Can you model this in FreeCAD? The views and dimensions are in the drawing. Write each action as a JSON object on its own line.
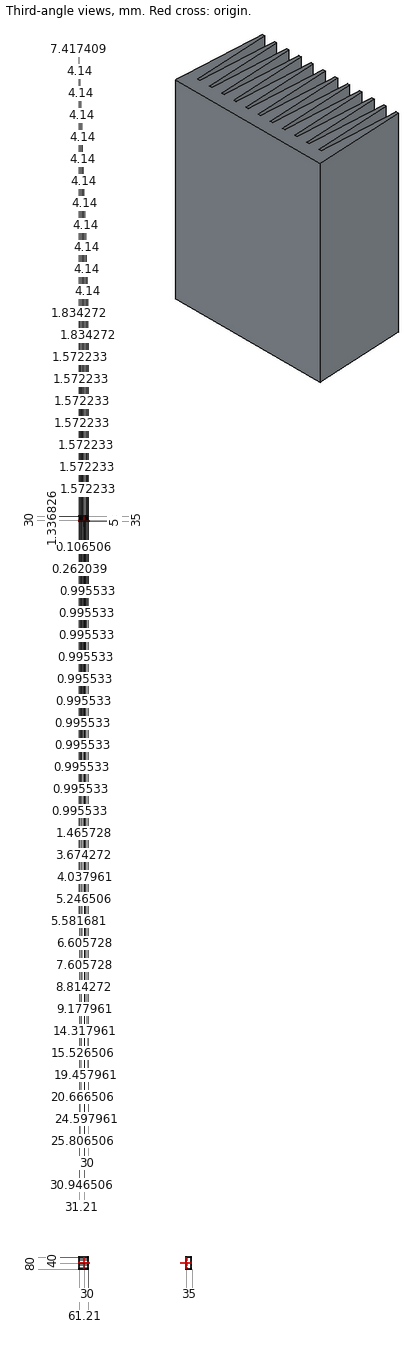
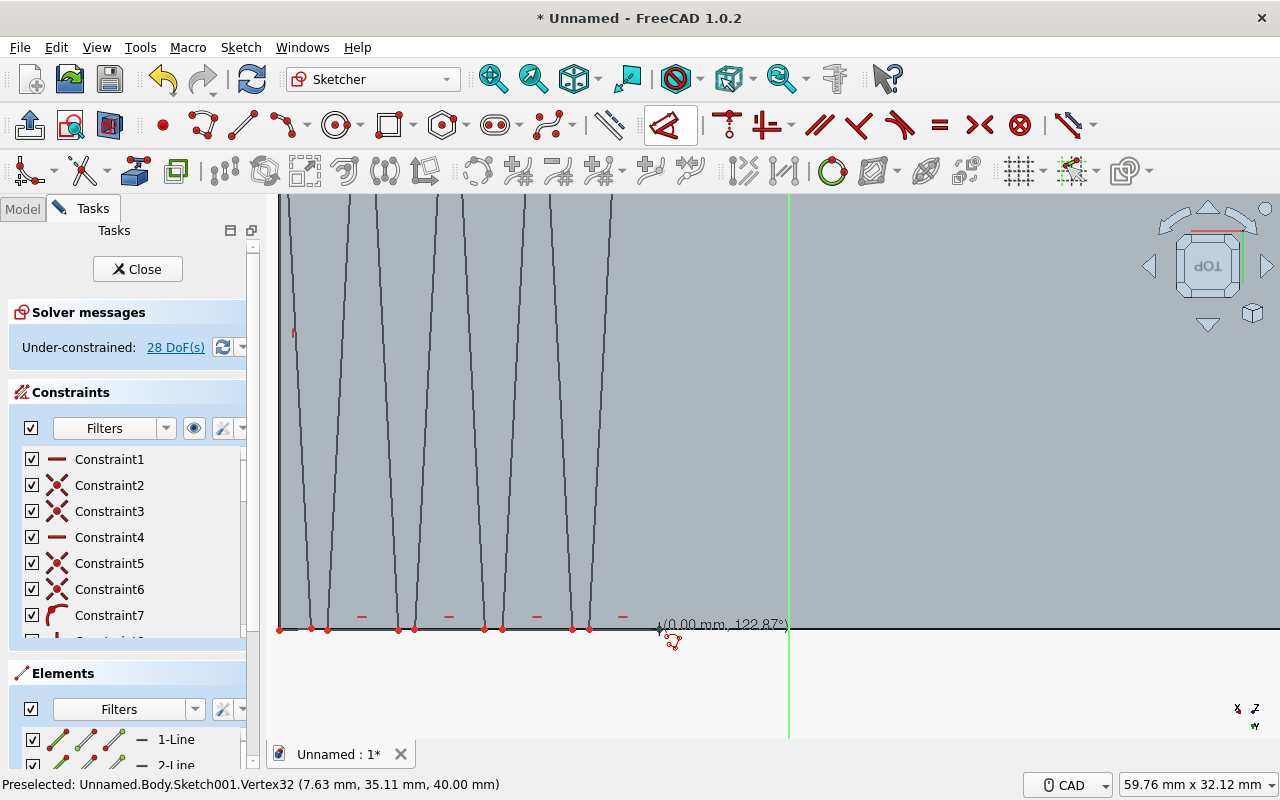
{"action": "scroll", "coordinate": [590, 630], "scroll_direction": "down", "scroll_amount": 3}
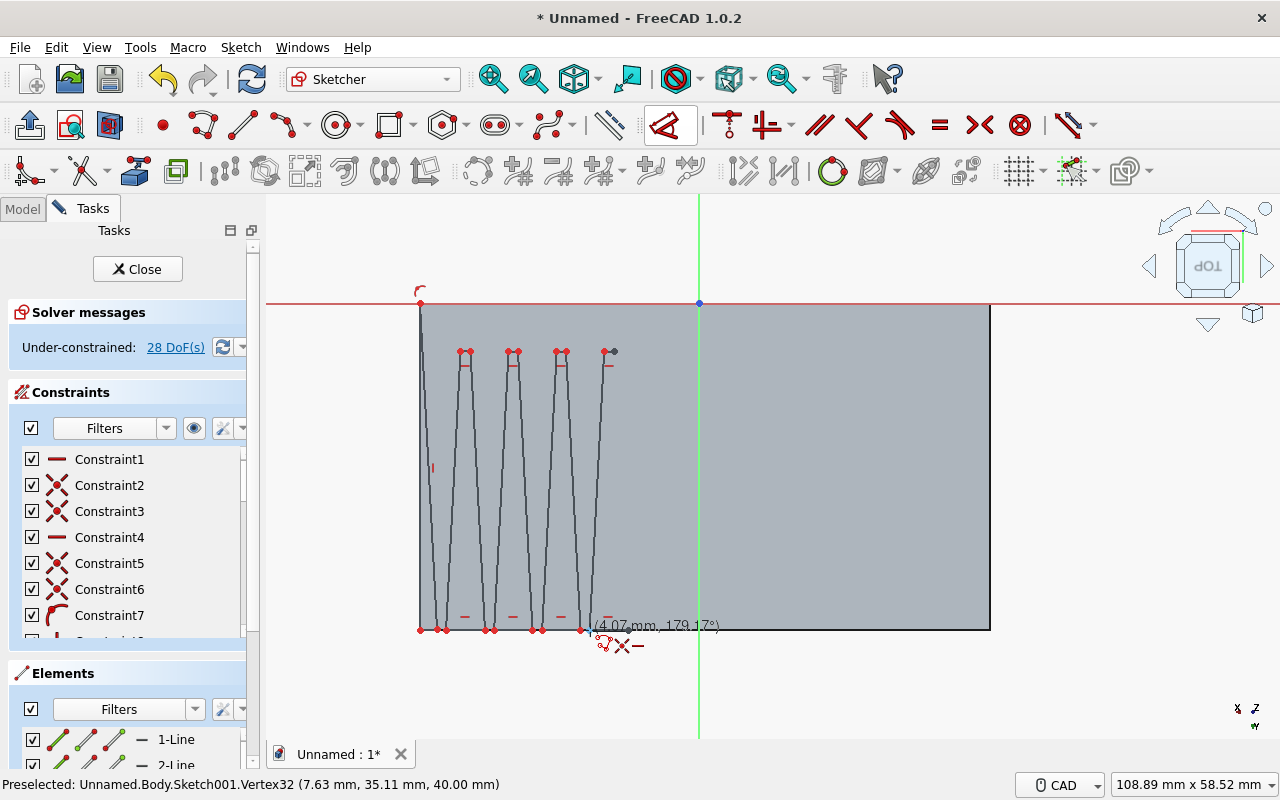
{"action": "scroll", "coordinate": [614, 351], "scroll_direction": "up", "scroll_amount": 7}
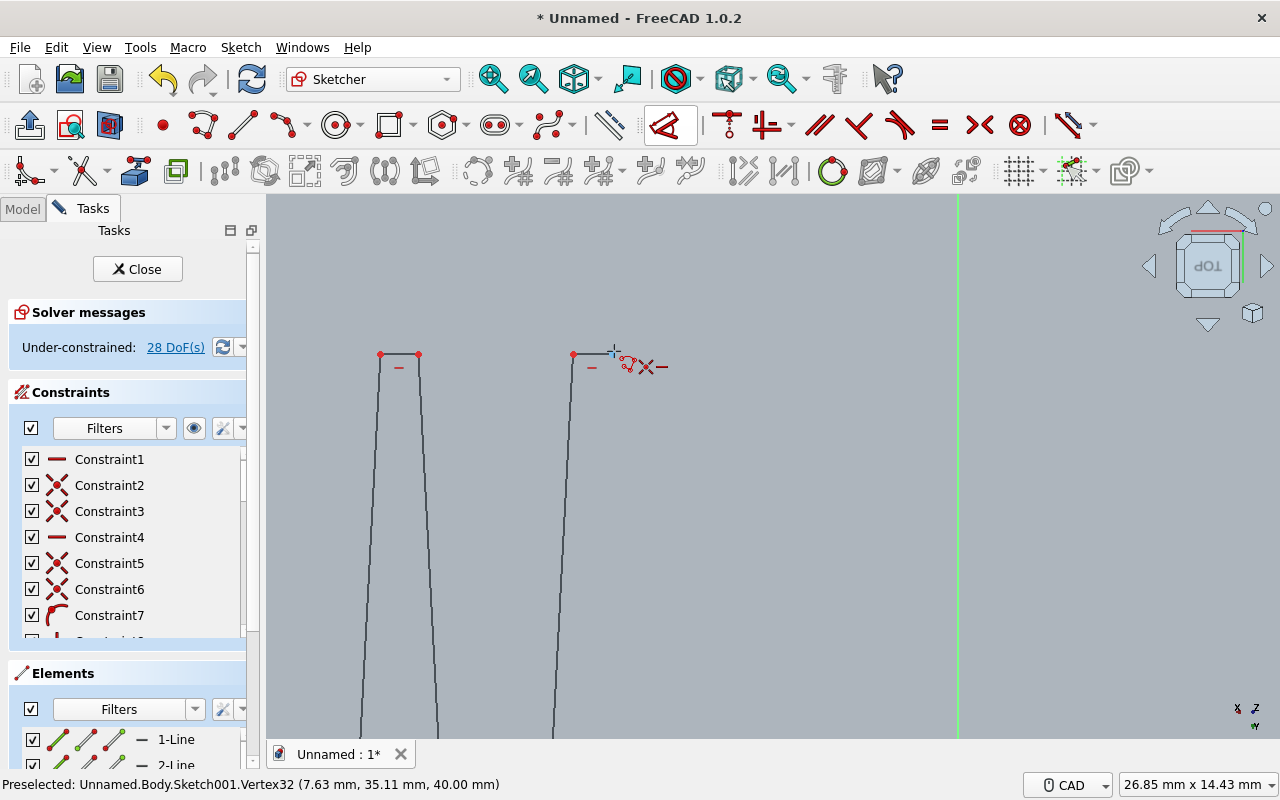
{"action": "left_click", "coordinate": [613, 354]}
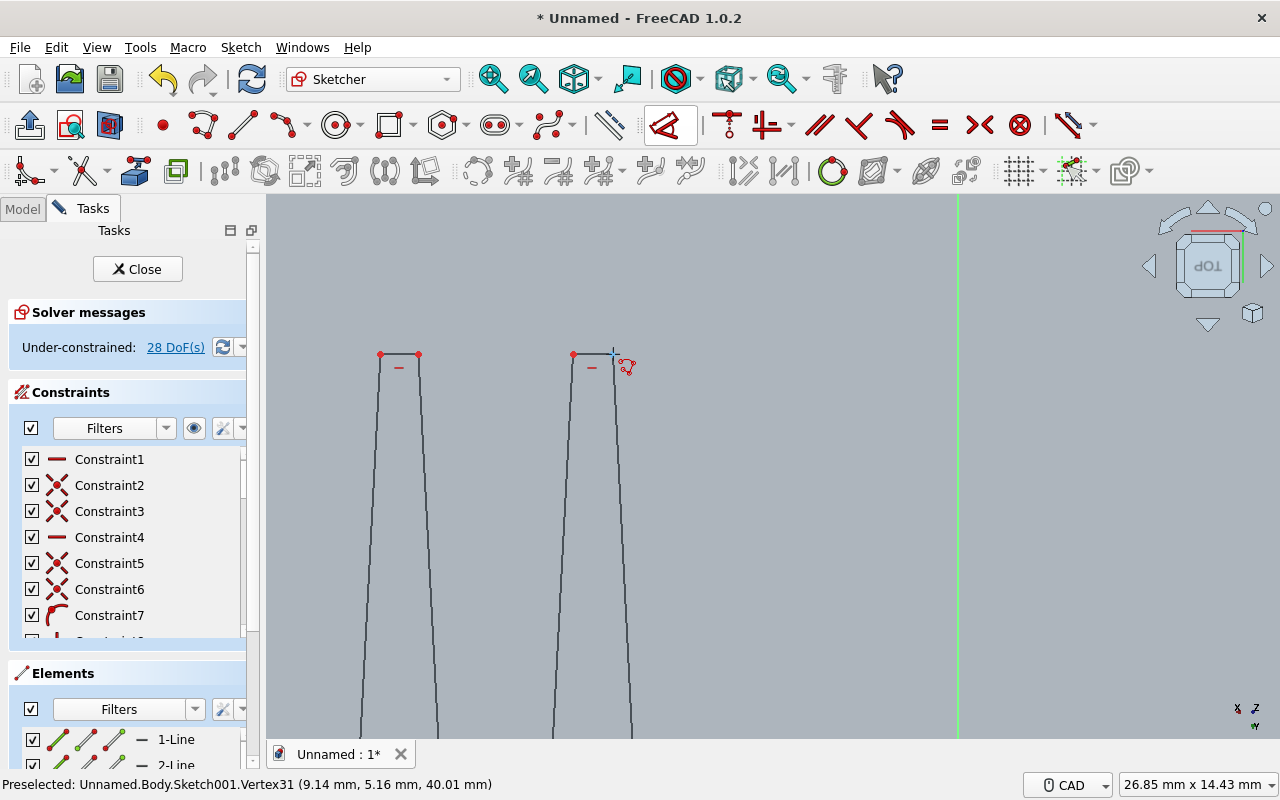
{"action": "scroll", "coordinate": [614, 351], "scroll_direction": "down", "scroll_amount": 7}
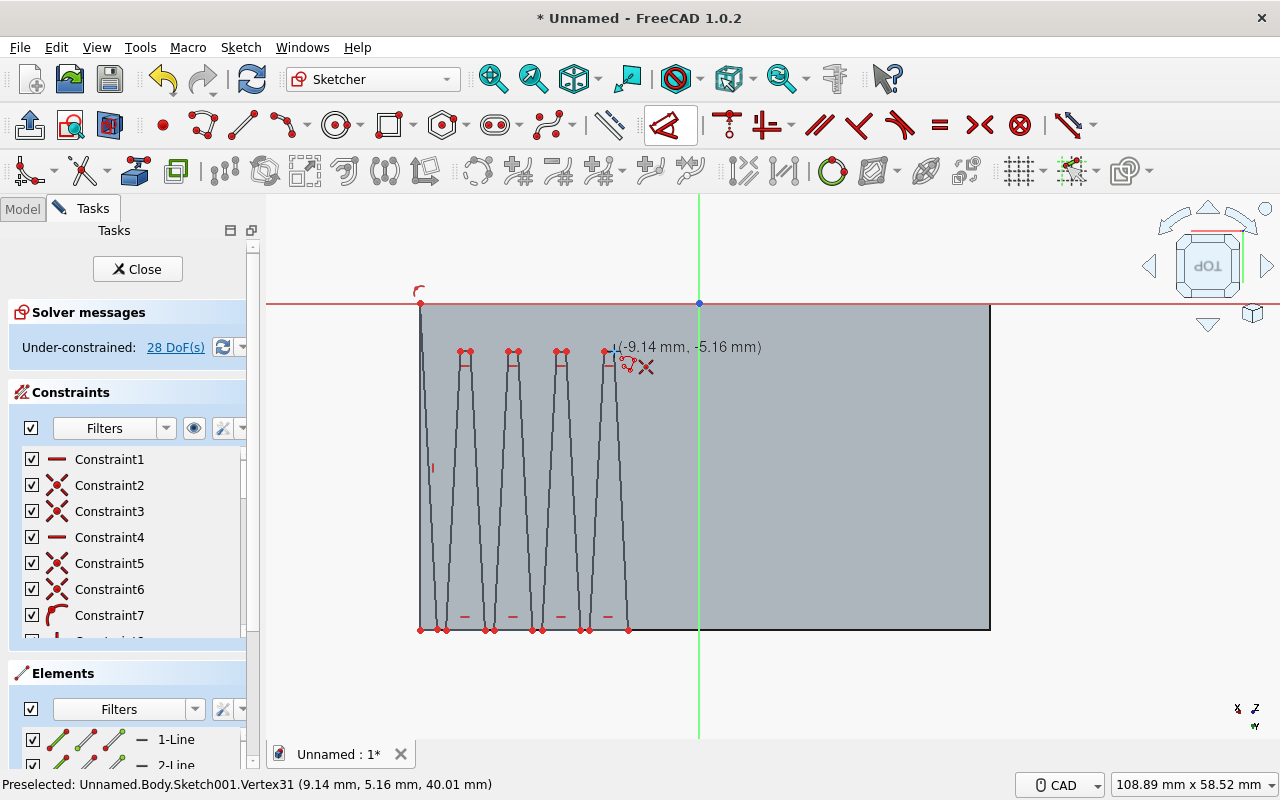
{"action": "left_click", "coordinate": [661, 351]}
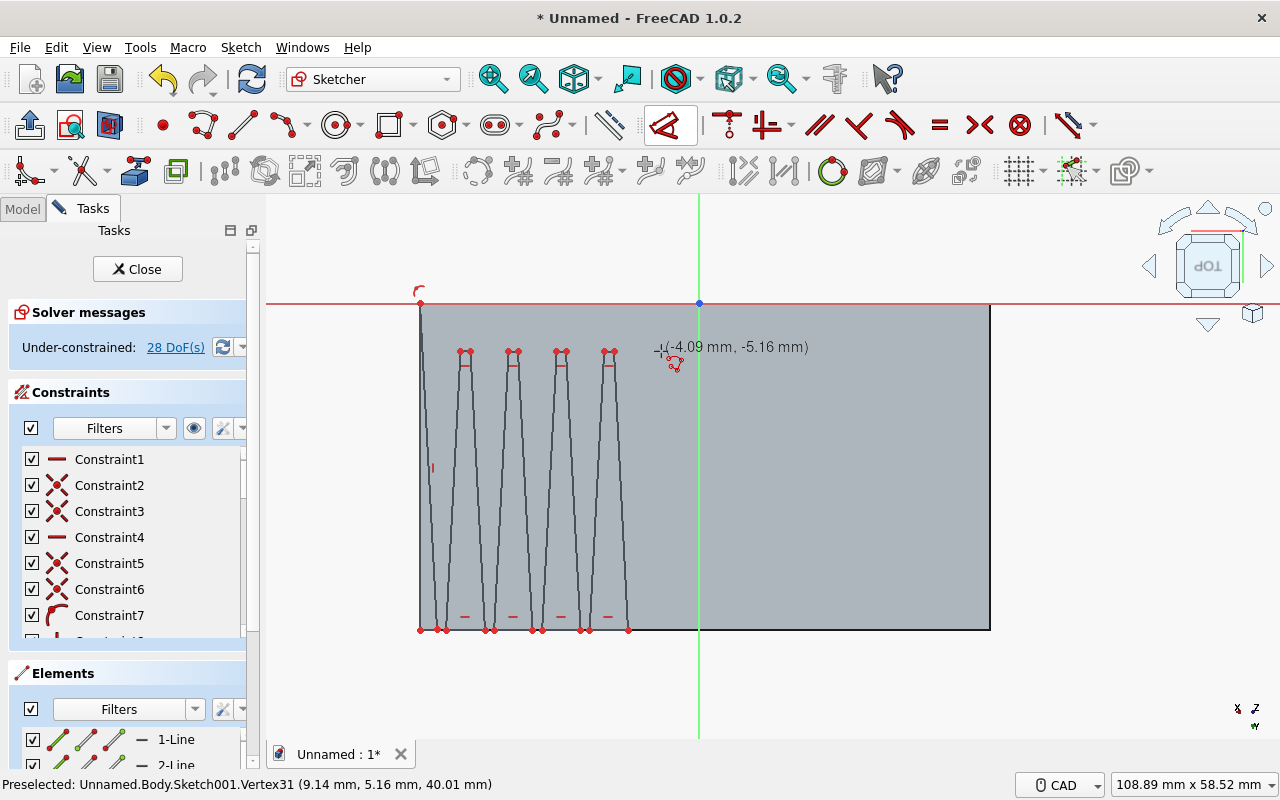
{"action": "scroll", "coordinate": [652, 351], "scroll_direction": "up", "scroll_amount": 3}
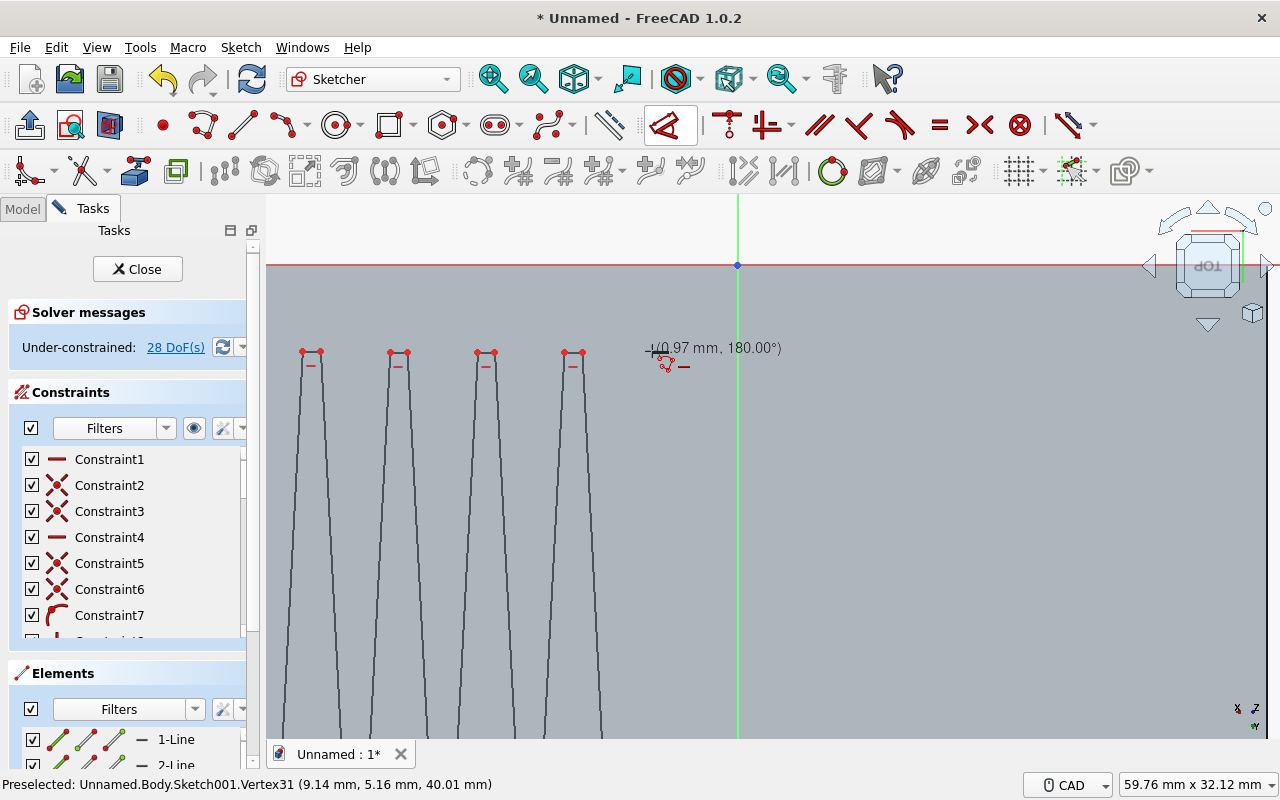
{"action": "left_click", "coordinate": [652, 351]}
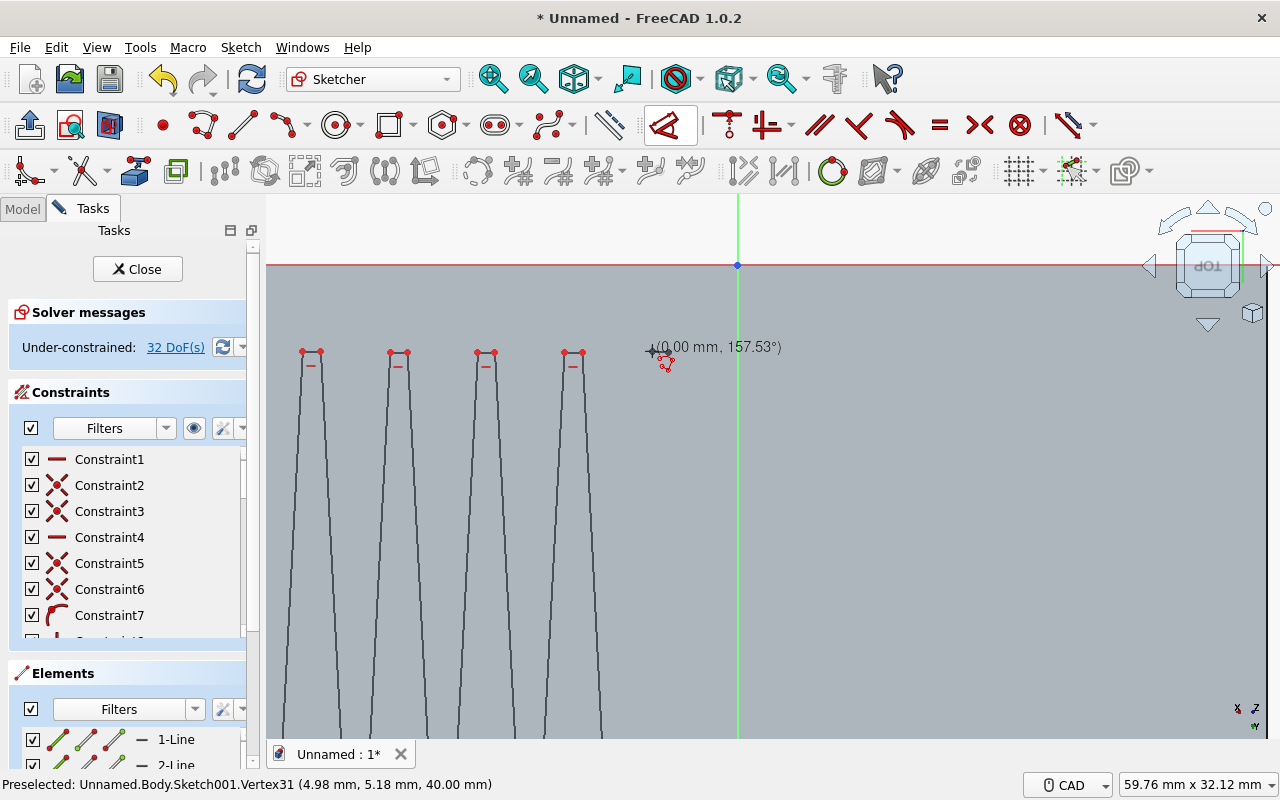
{"action": "scroll", "coordinate": [652, 350], "scroll_direction": "down", "scroll_amount": 3}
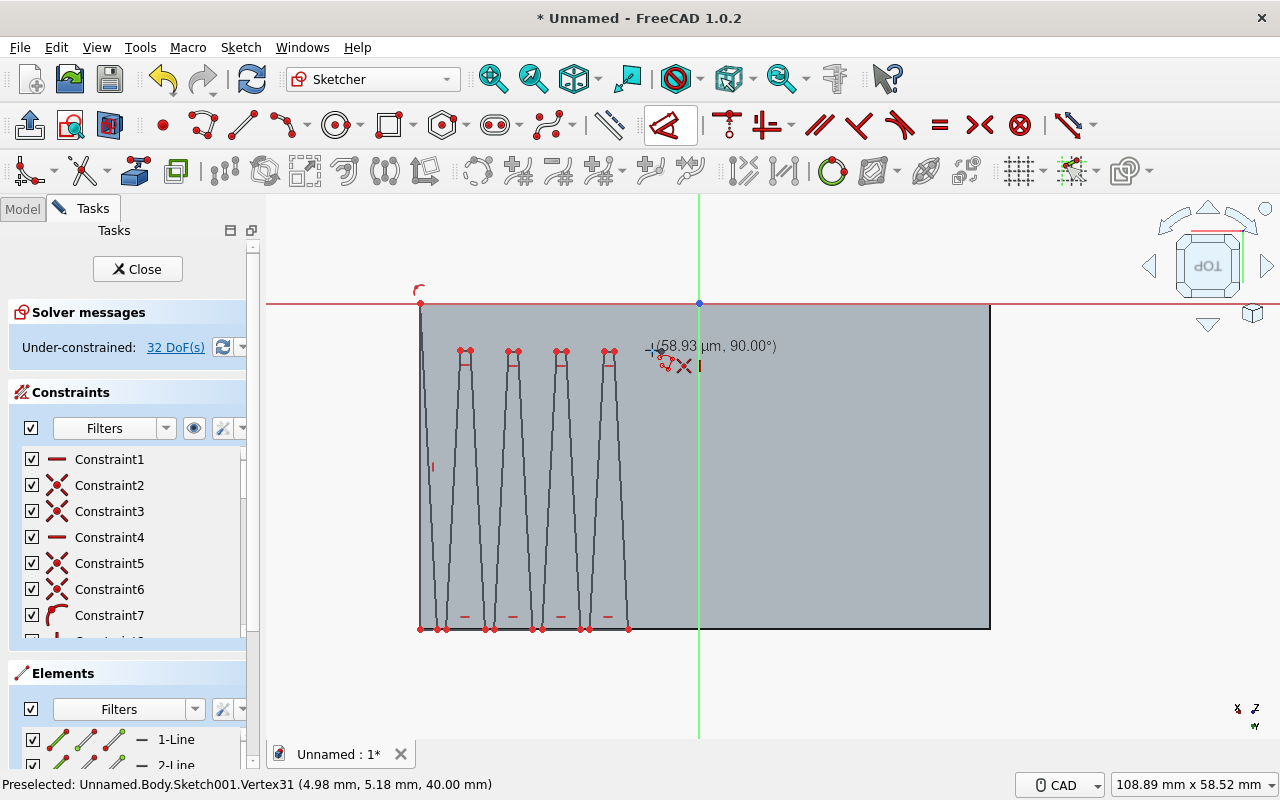
{"action": "scroll", "coordinate": [638, 629], "scroll_direction": "up", "scroll_amount": 3}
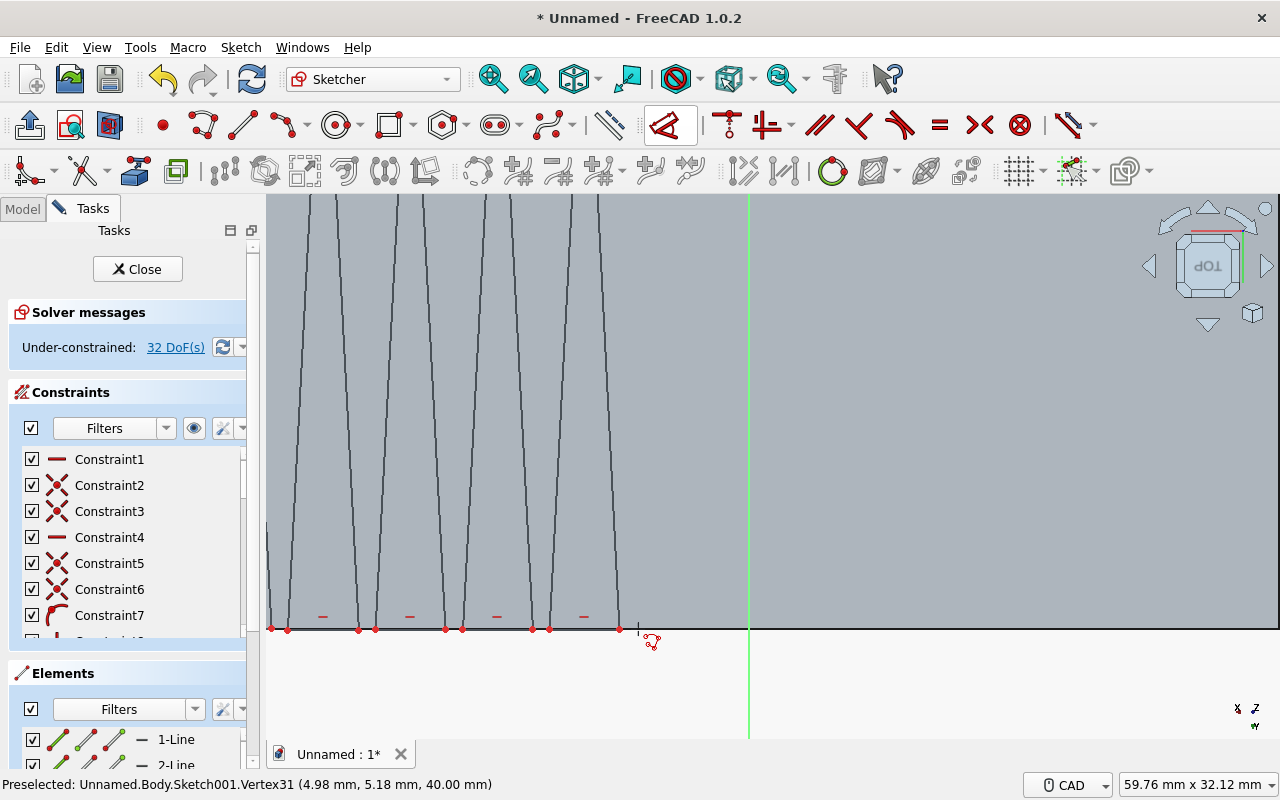
{"action": "left_click", "coordinate": [637, 629]}
{"action": "left_click", "coordinate": [707, 629]}